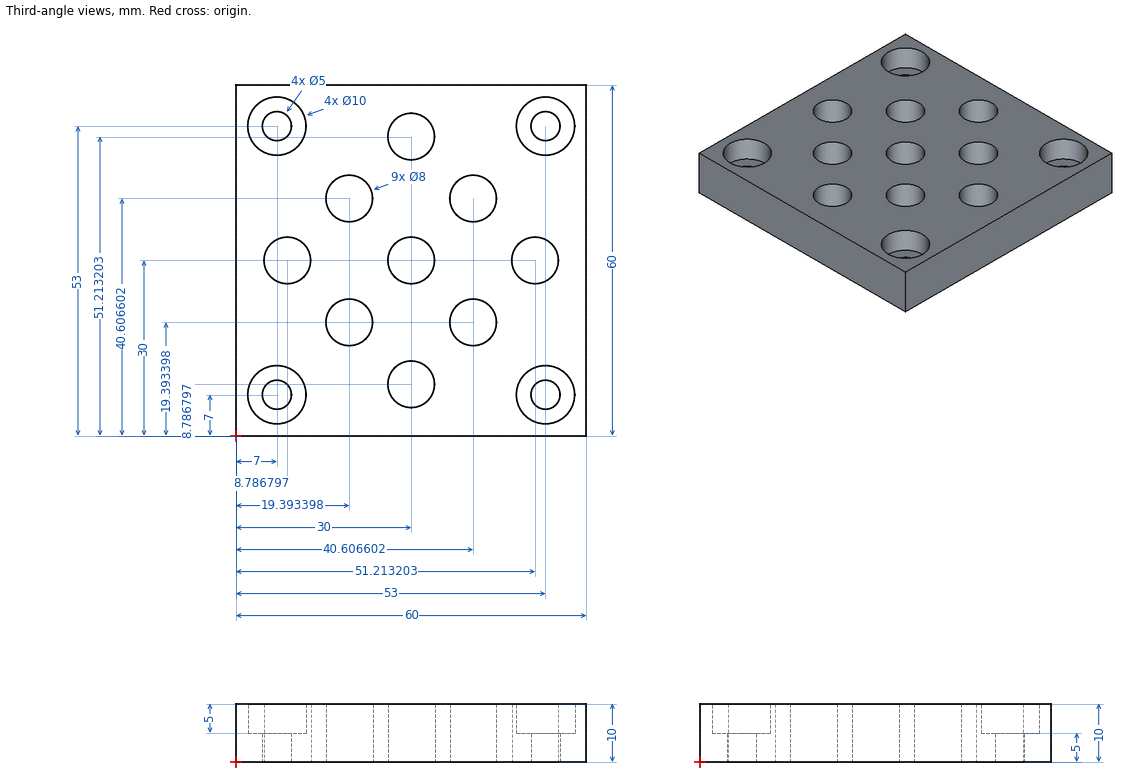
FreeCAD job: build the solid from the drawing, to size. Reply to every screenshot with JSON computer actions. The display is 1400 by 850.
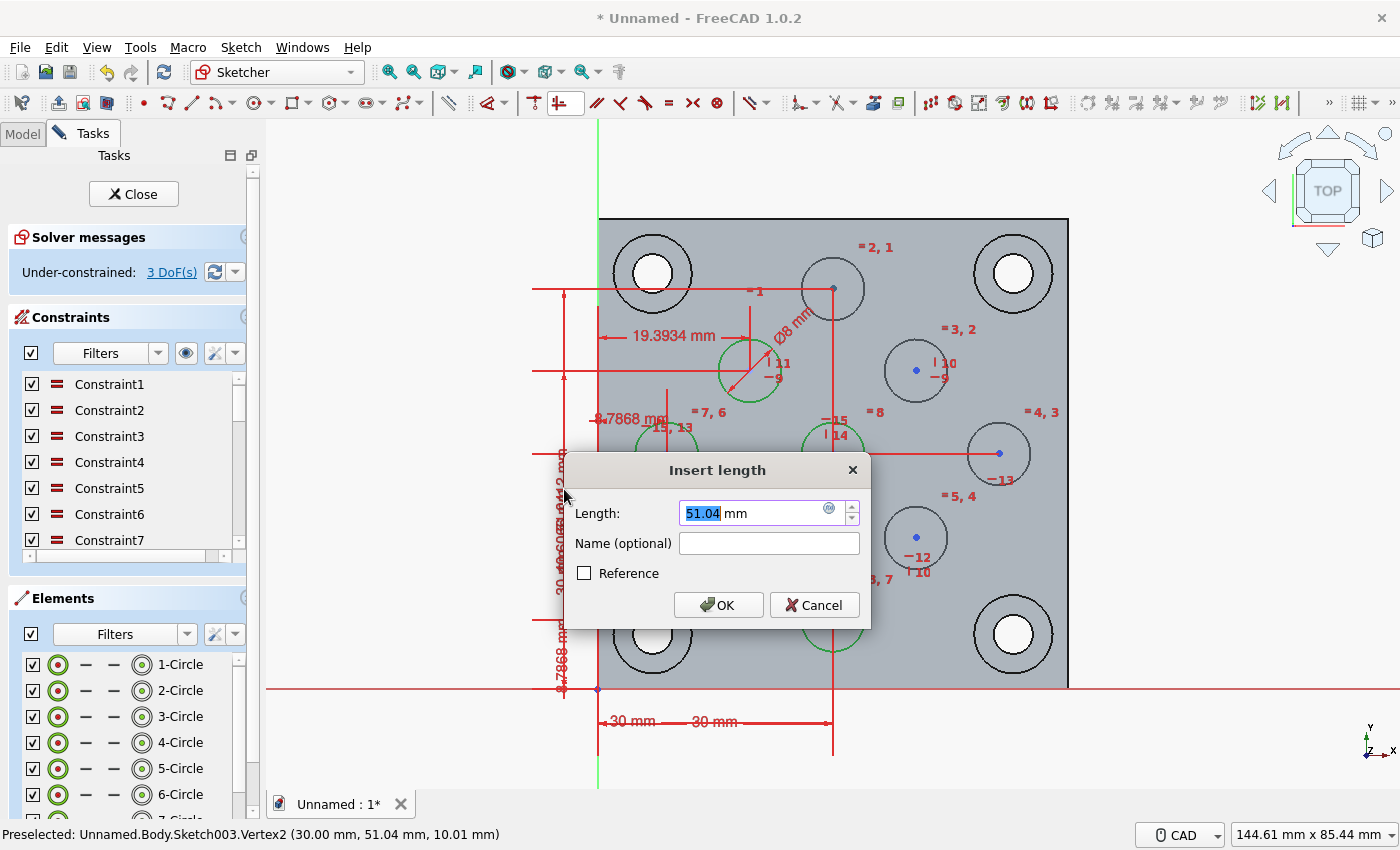
{"action": "type", "text": "51.213203"}
{"action": "key", "text": "Return"}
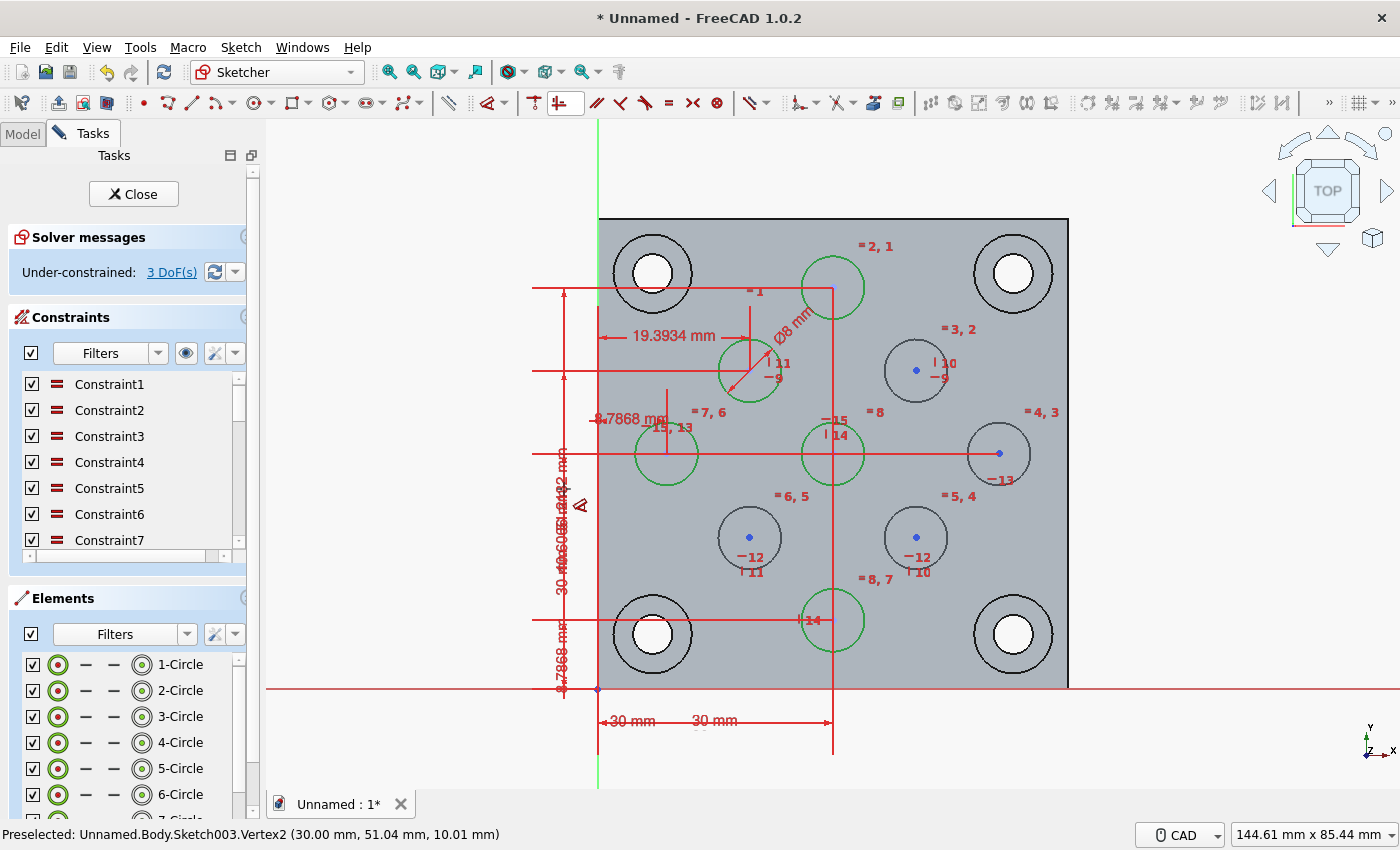
{"action": "left_click", "coordinate": [916, 371]}
{"action": "left_click", "coordinate": [830, 723]}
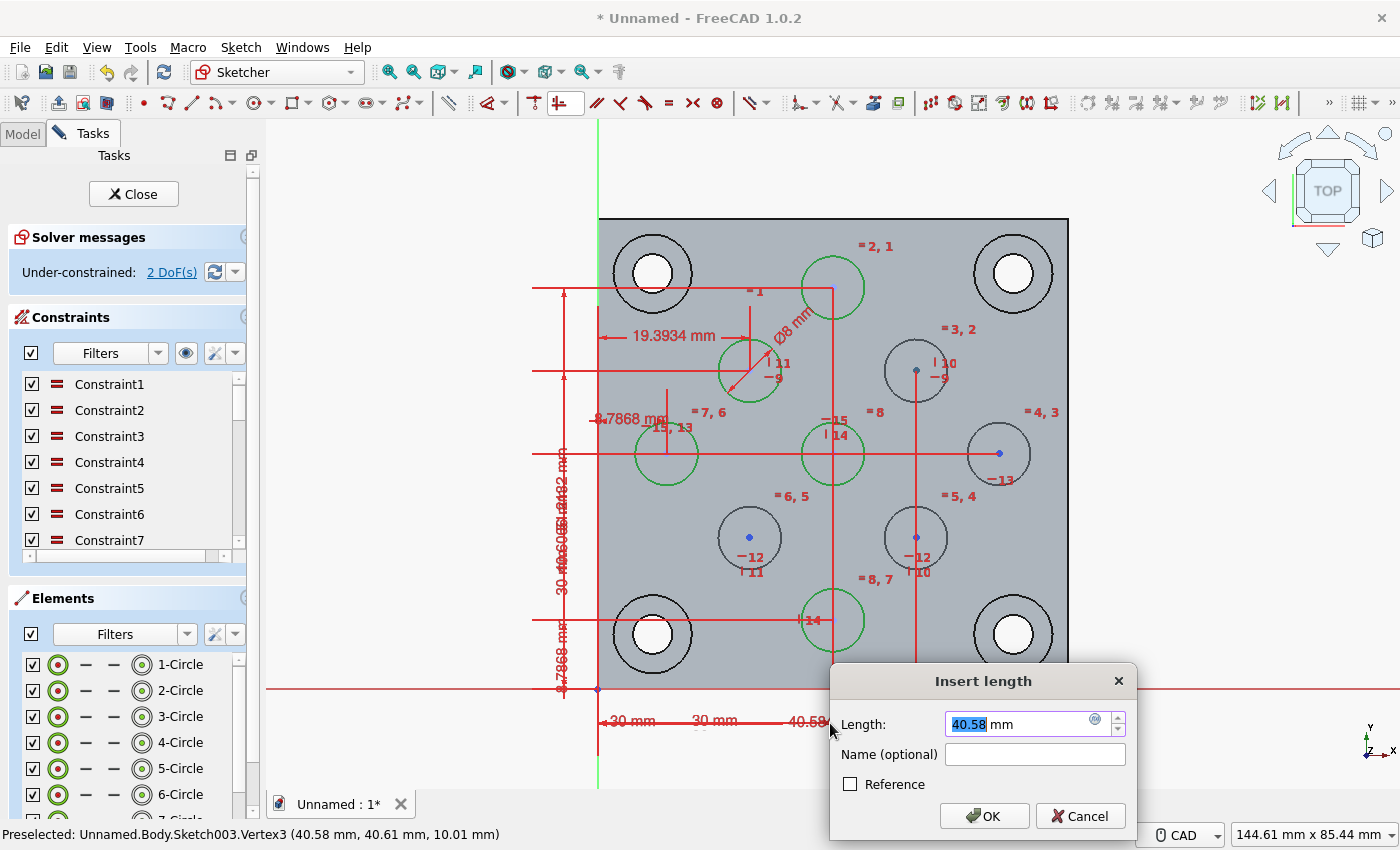
{"action": "type", "text": "40.606602"}
{"action": "key", "text": "Return"}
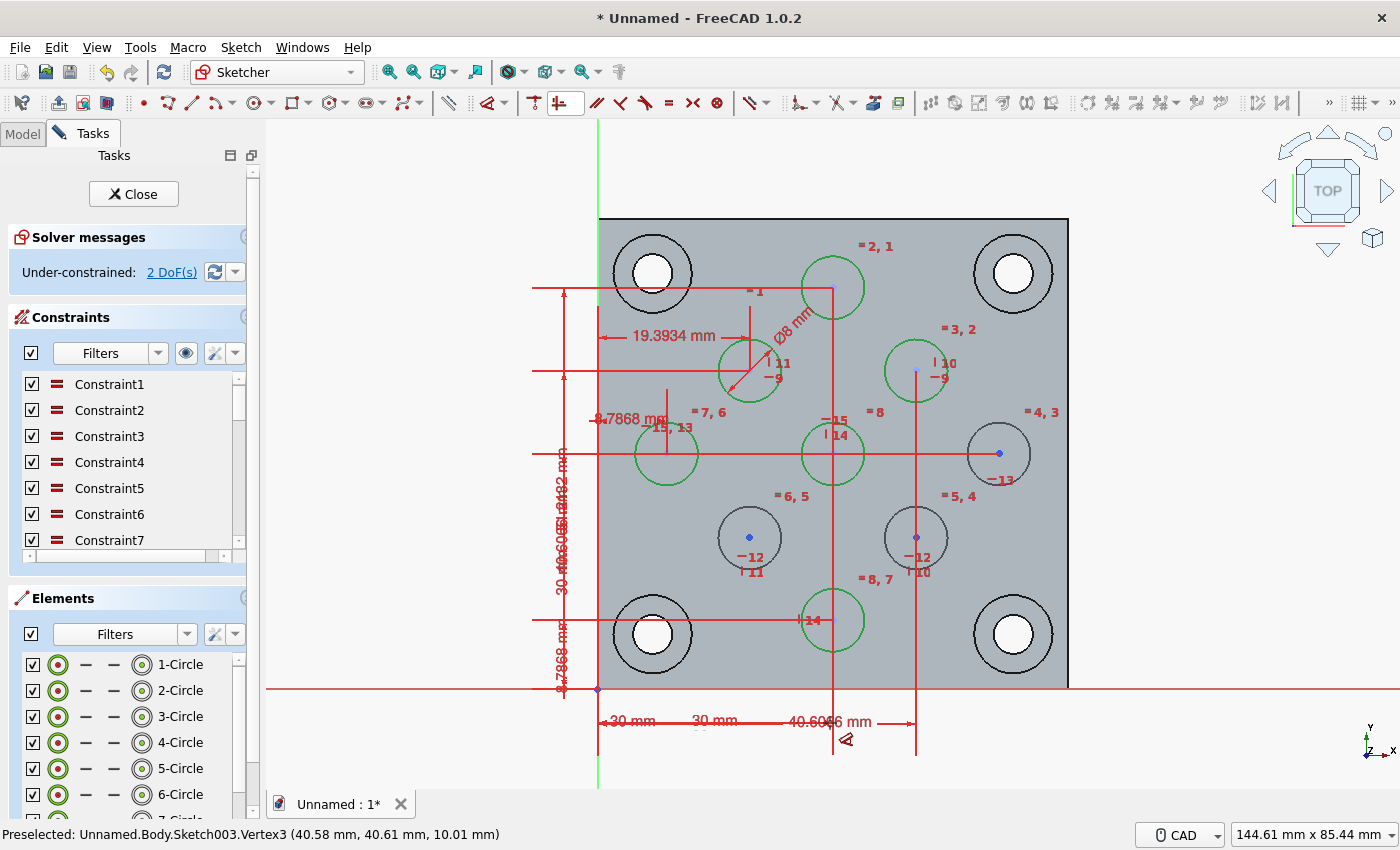
{"action": "left_click", "coordinate": [999, 454]}
{"action": "left_click", "coordinate": [939, 723]}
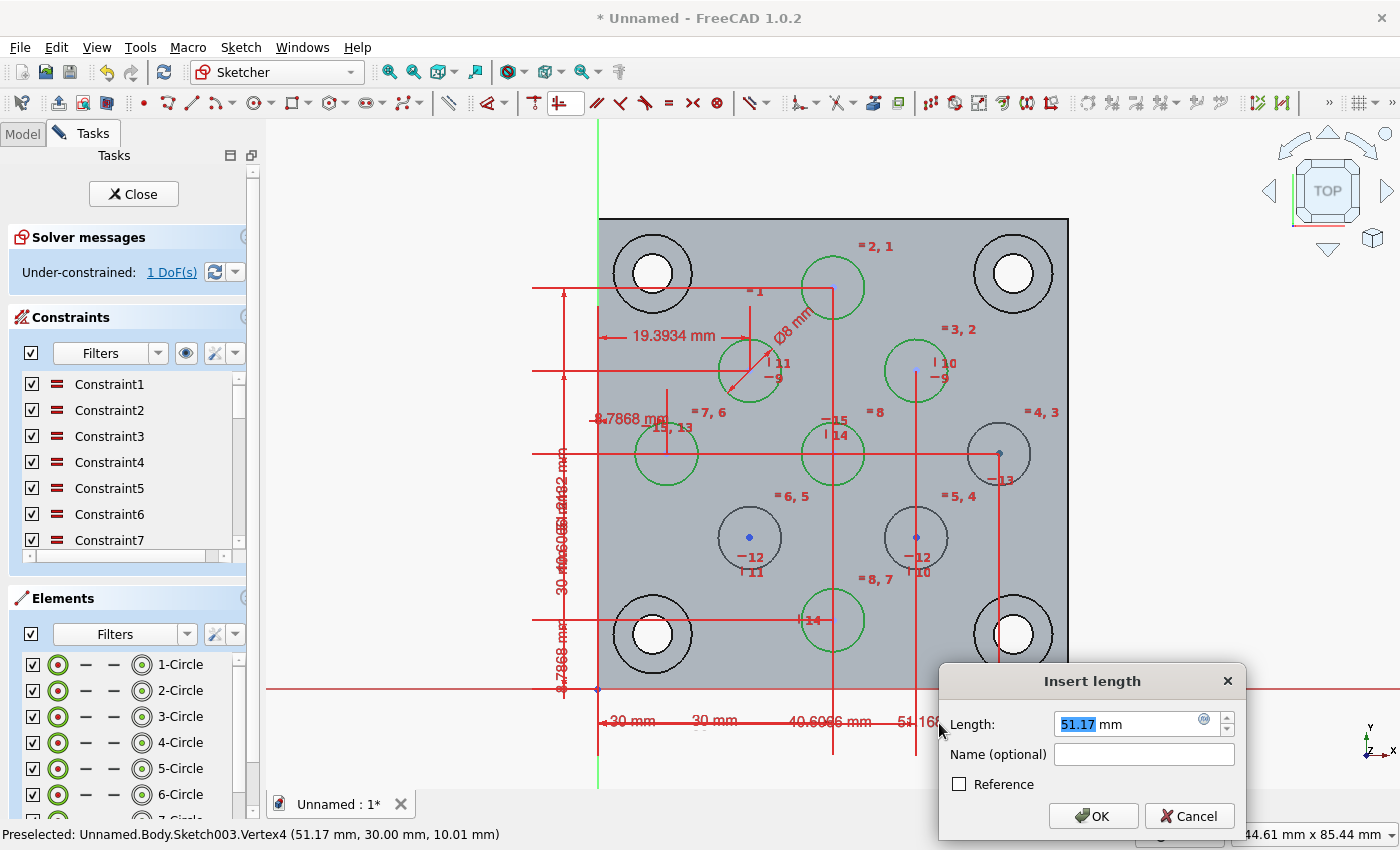
{"action": "type", "text": "51.213203"}
{"action": "key", "text": "Return"}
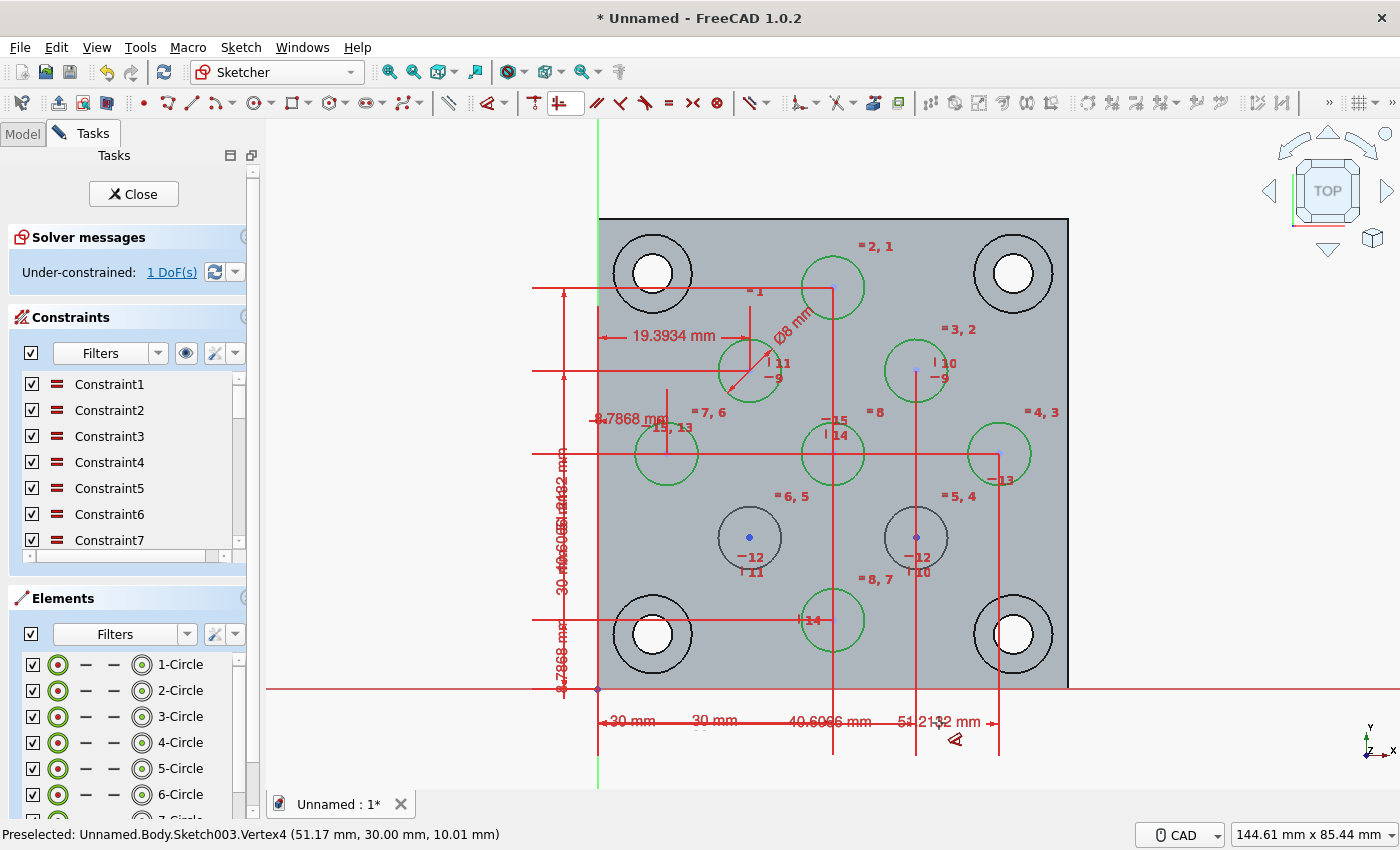
{"action": "left_click", "coordinate": [916, 538]}
{"action": "left_click", "coordinate": [564, 614]}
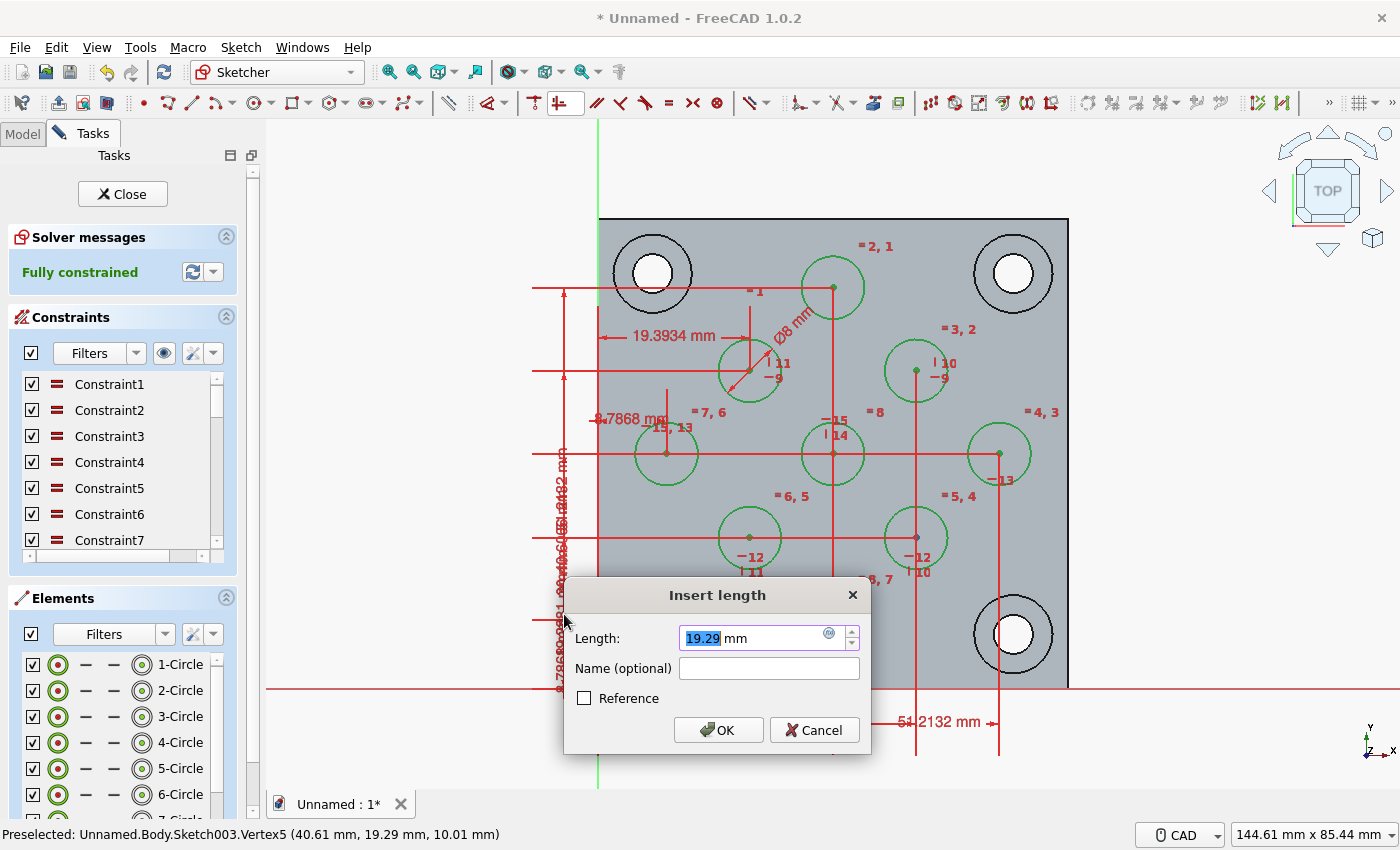
{"action": "type", "text": "19.393398"}
{"action": "key", "text": "Return"}
{"action": "key", "text": "Escape"}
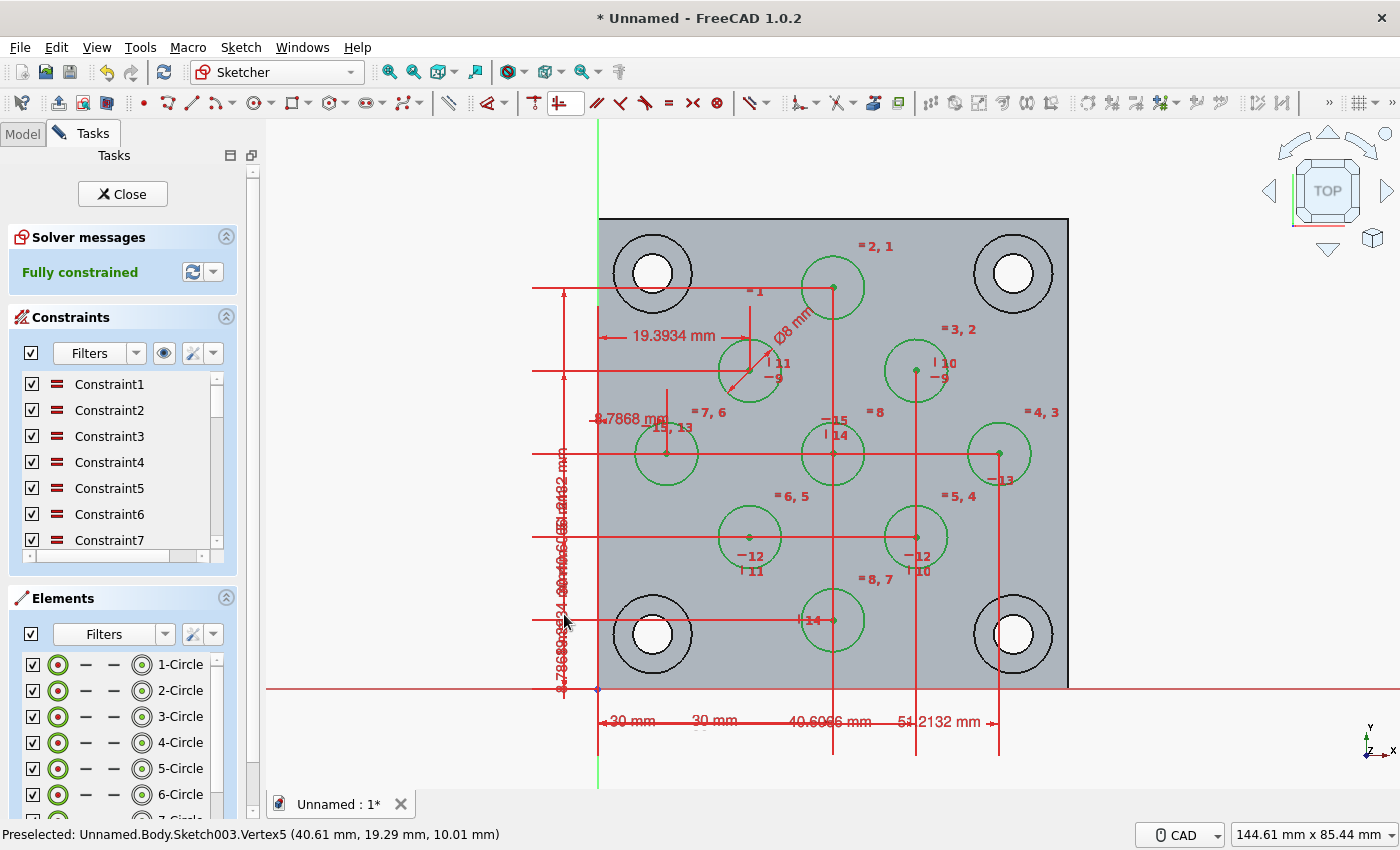
{"action": "left_click", "coordinate": [123, 194]}